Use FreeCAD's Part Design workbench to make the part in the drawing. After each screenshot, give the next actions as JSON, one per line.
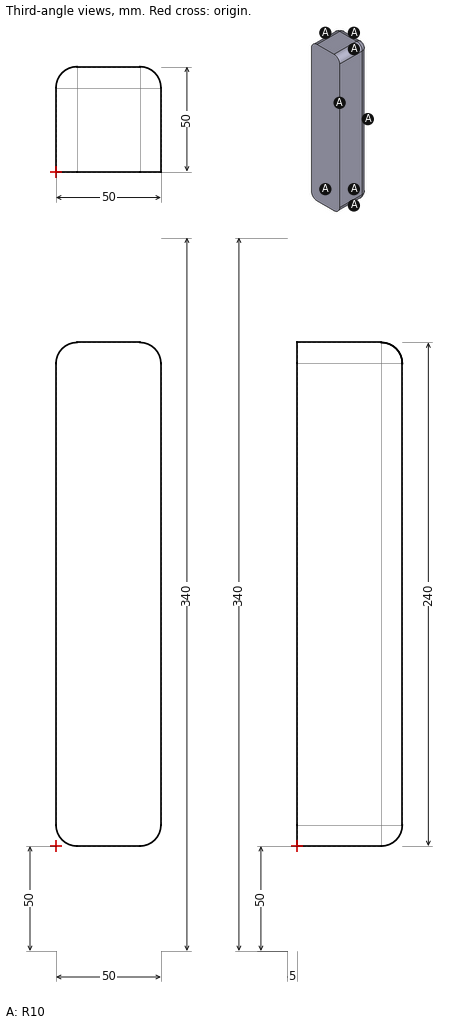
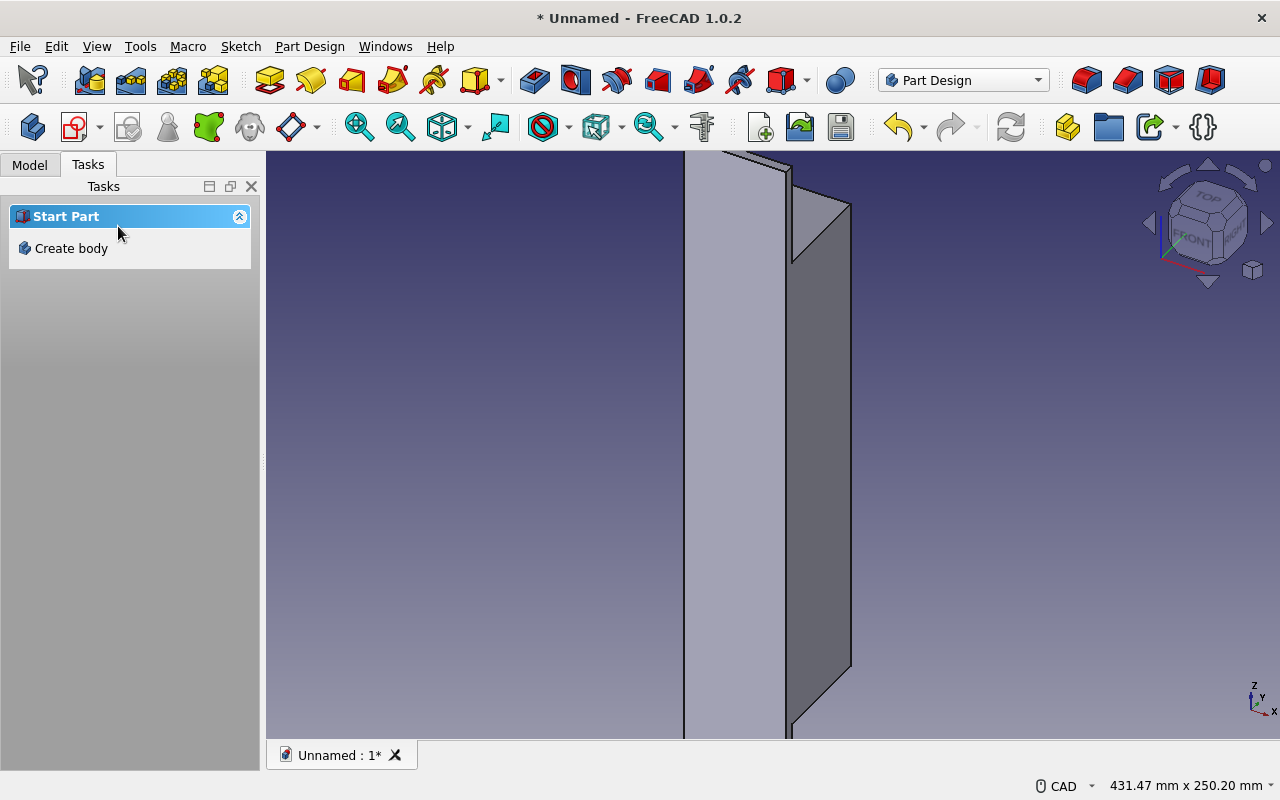
{"action": "left_click", "coordinate": [360, 128]}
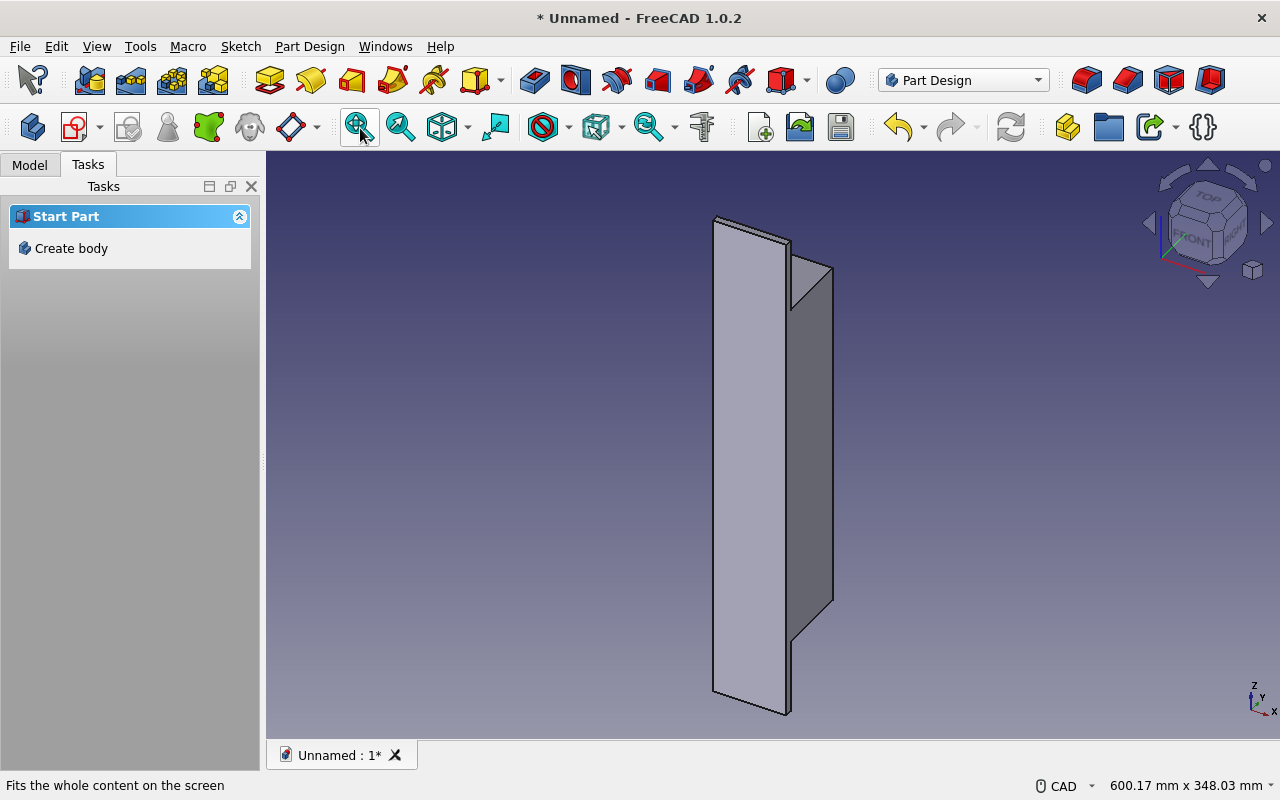
{"action": "left_click", "coordinate": [812, 288]}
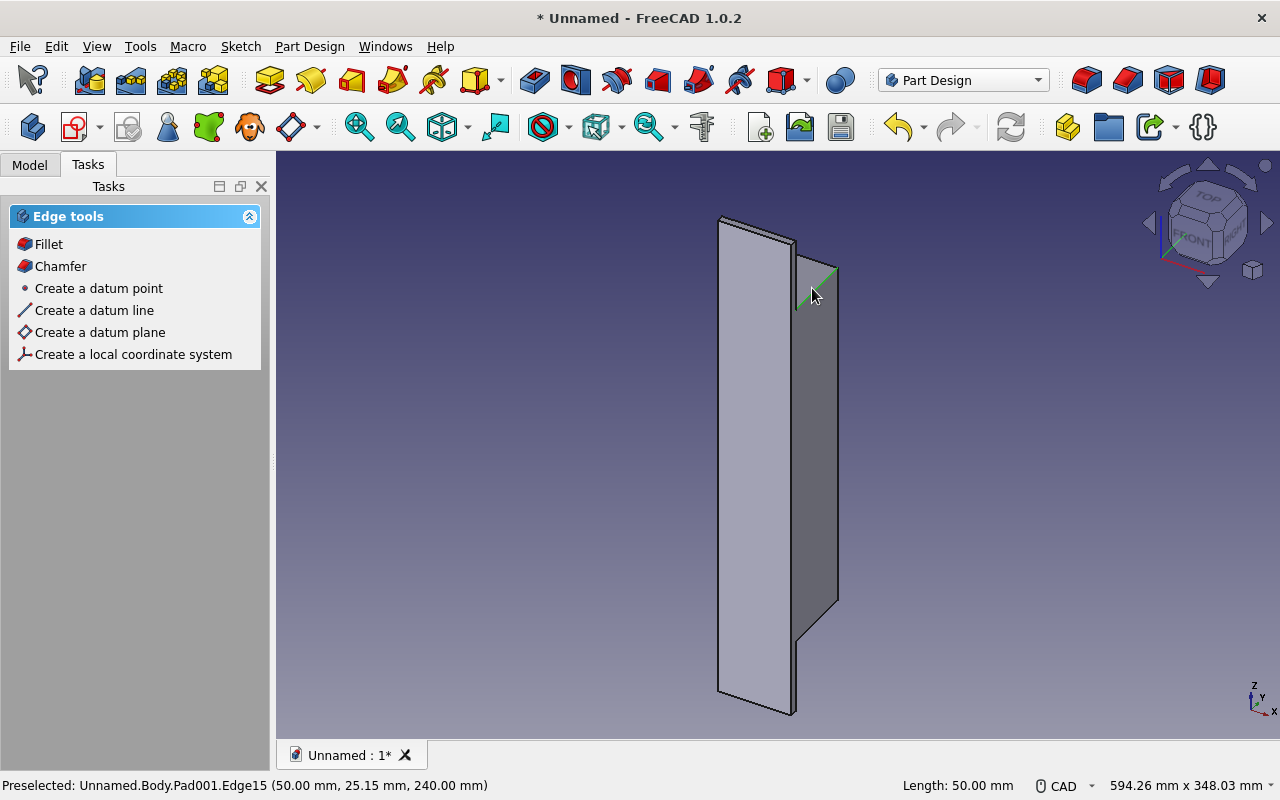
{"action": "key", "text": "0"}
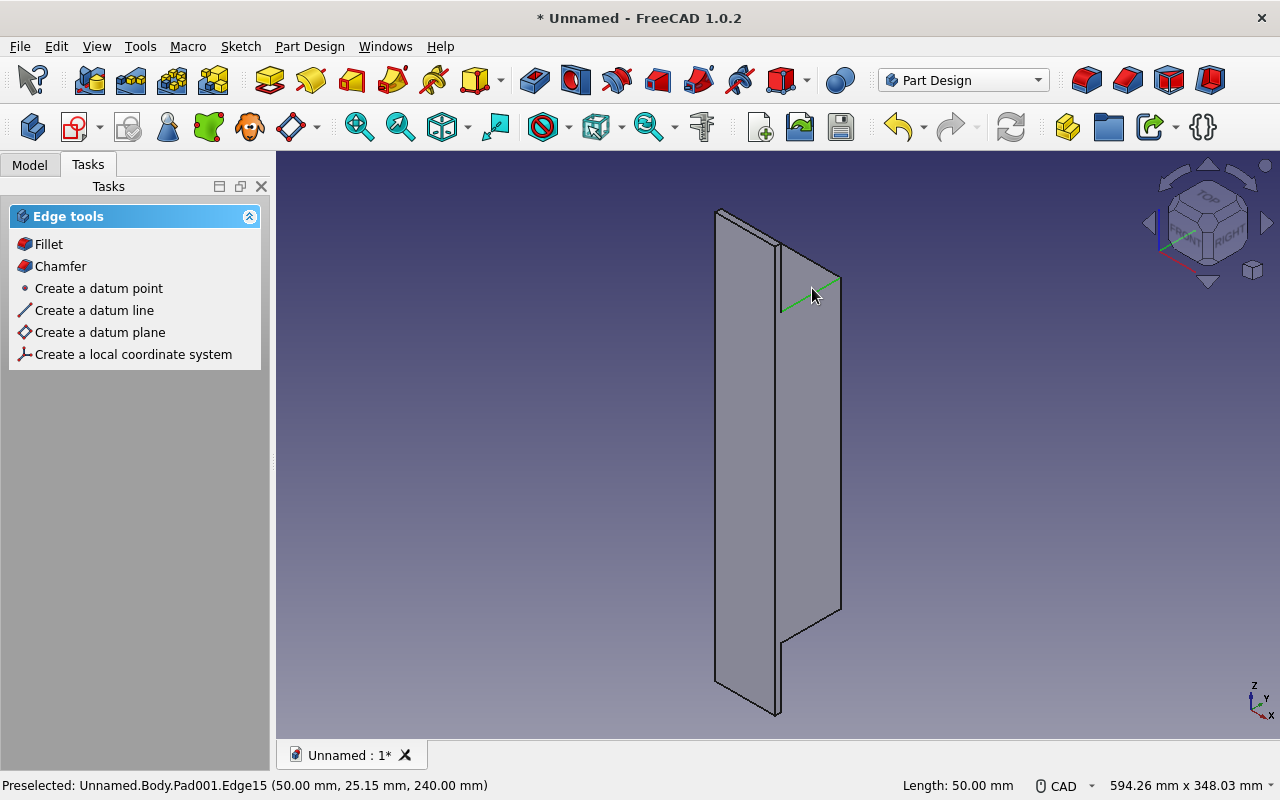
{"action": "key", "text": "2"}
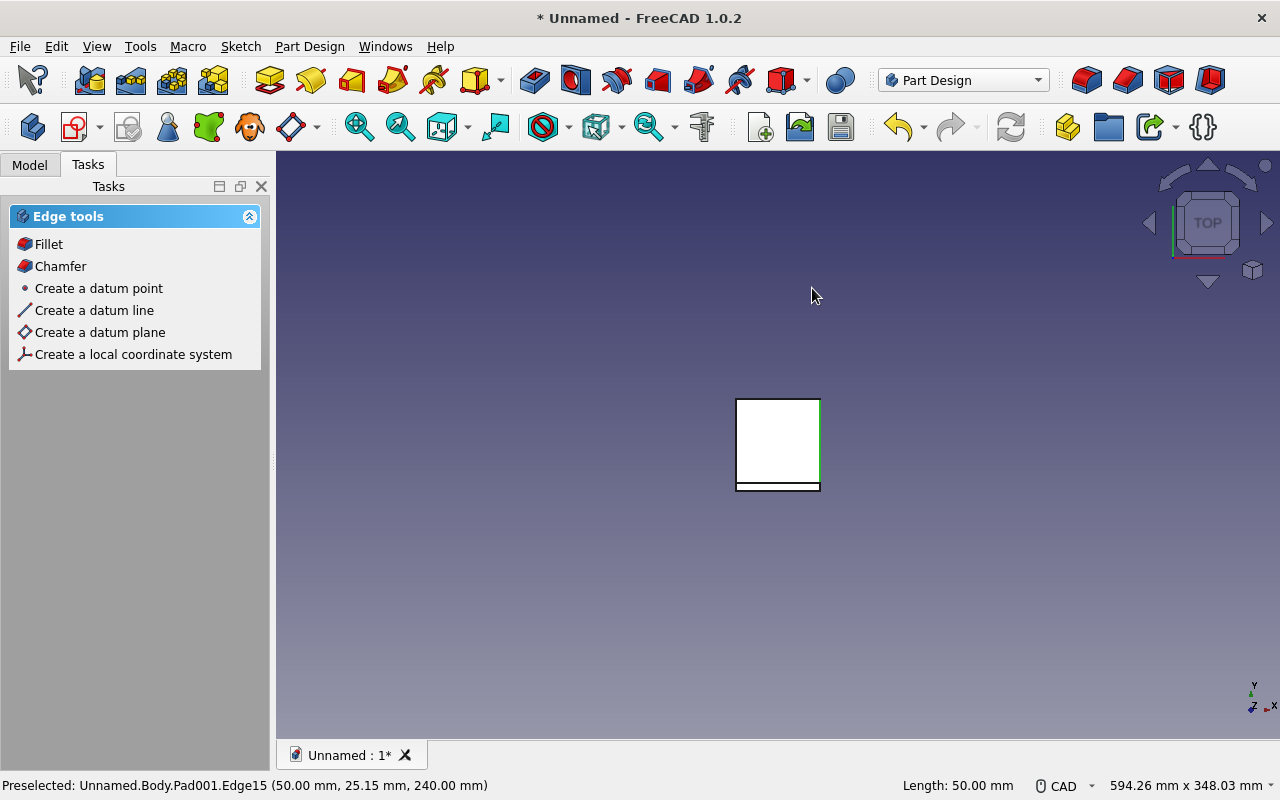
{"action": "left_click", "coordinate": [360, 128]}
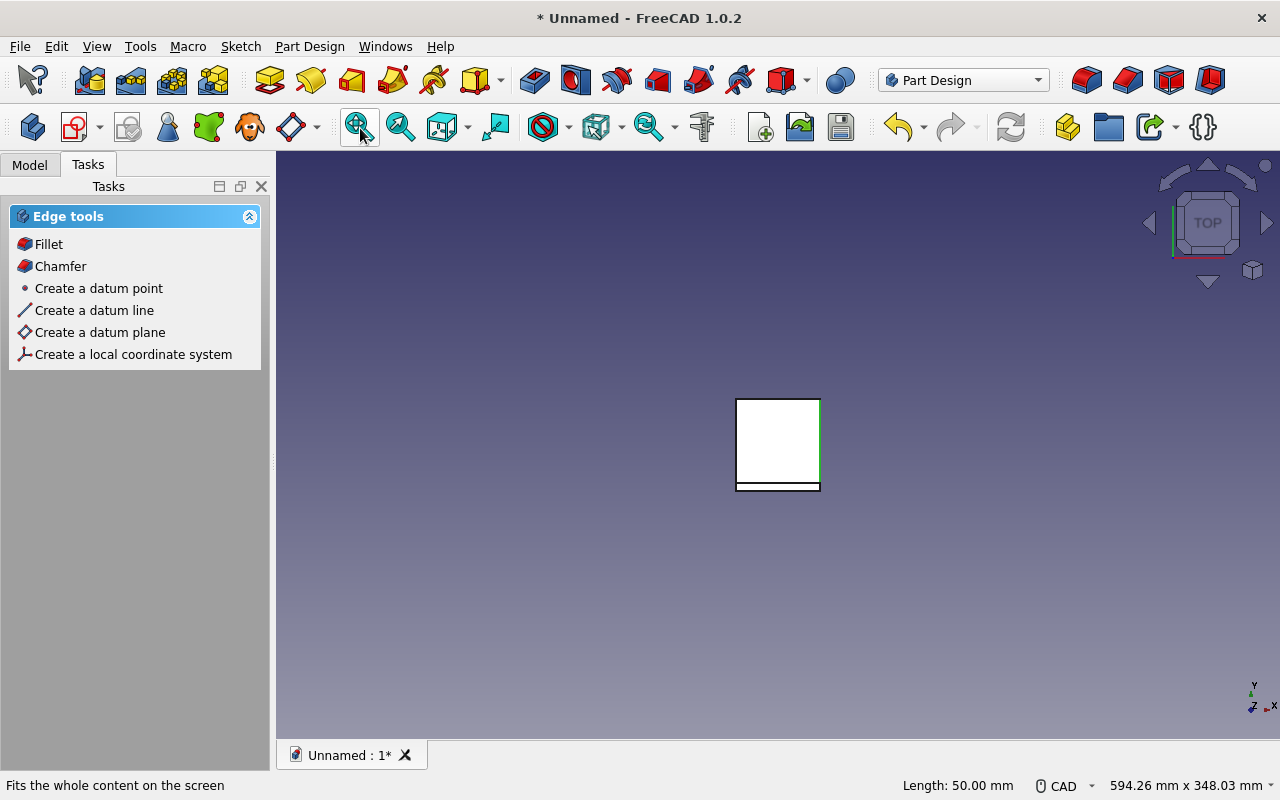
{"action": "left_click", "coordinate": [736, 440], "text": "ctrl"}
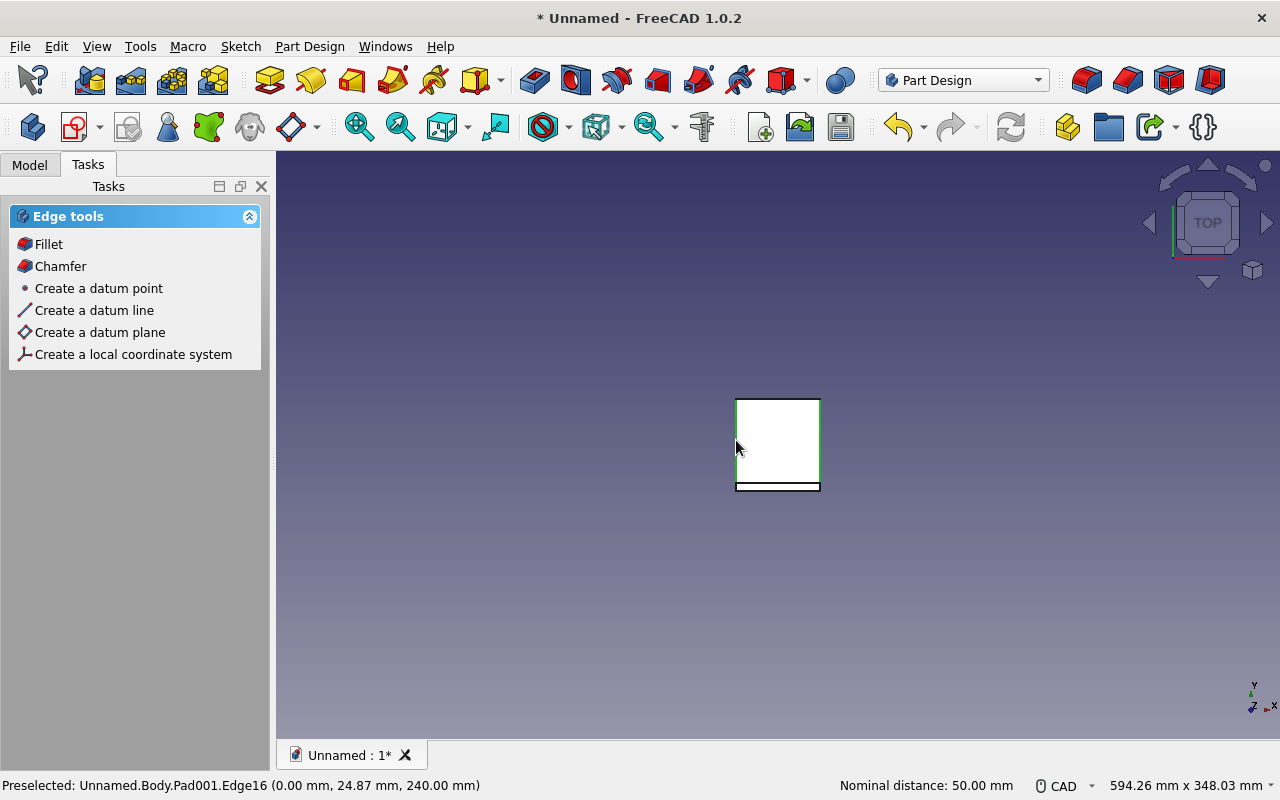
{"action": "key", "text": "1"}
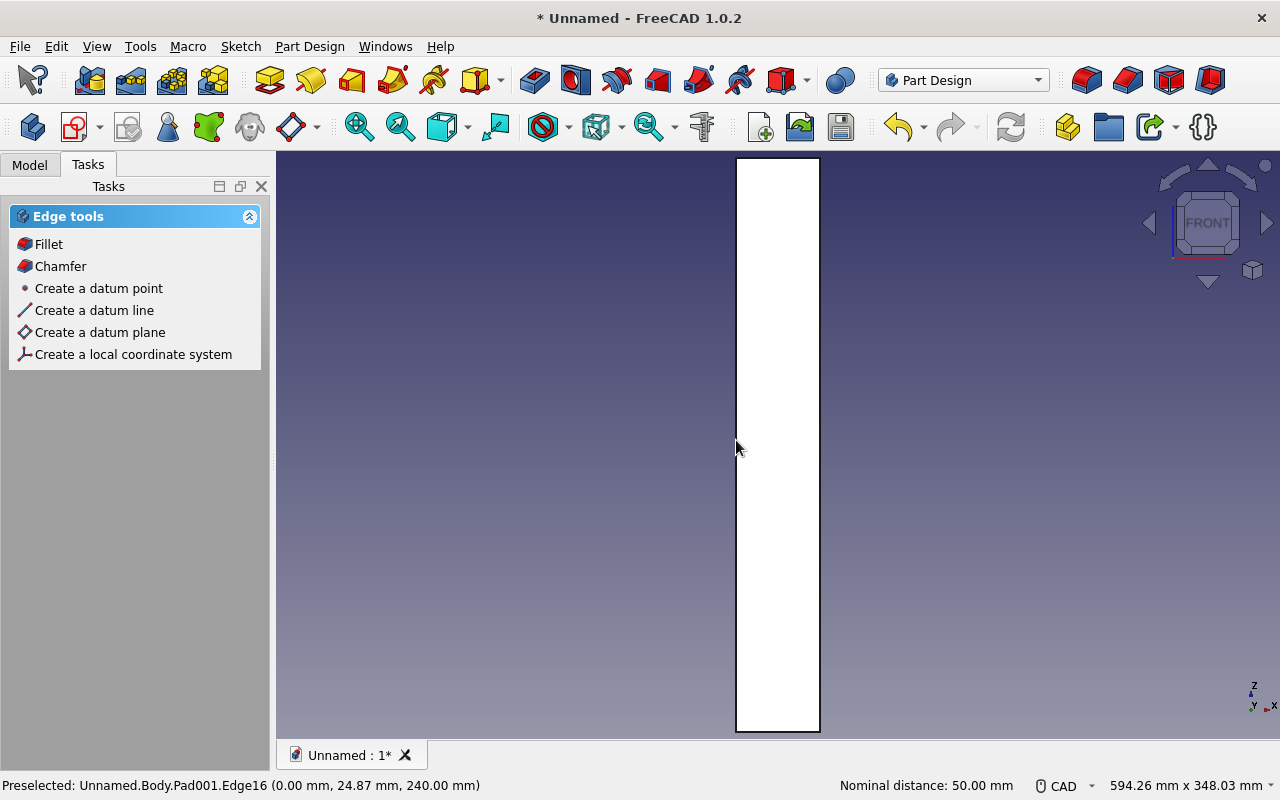
{"action": "key", "text": "3"}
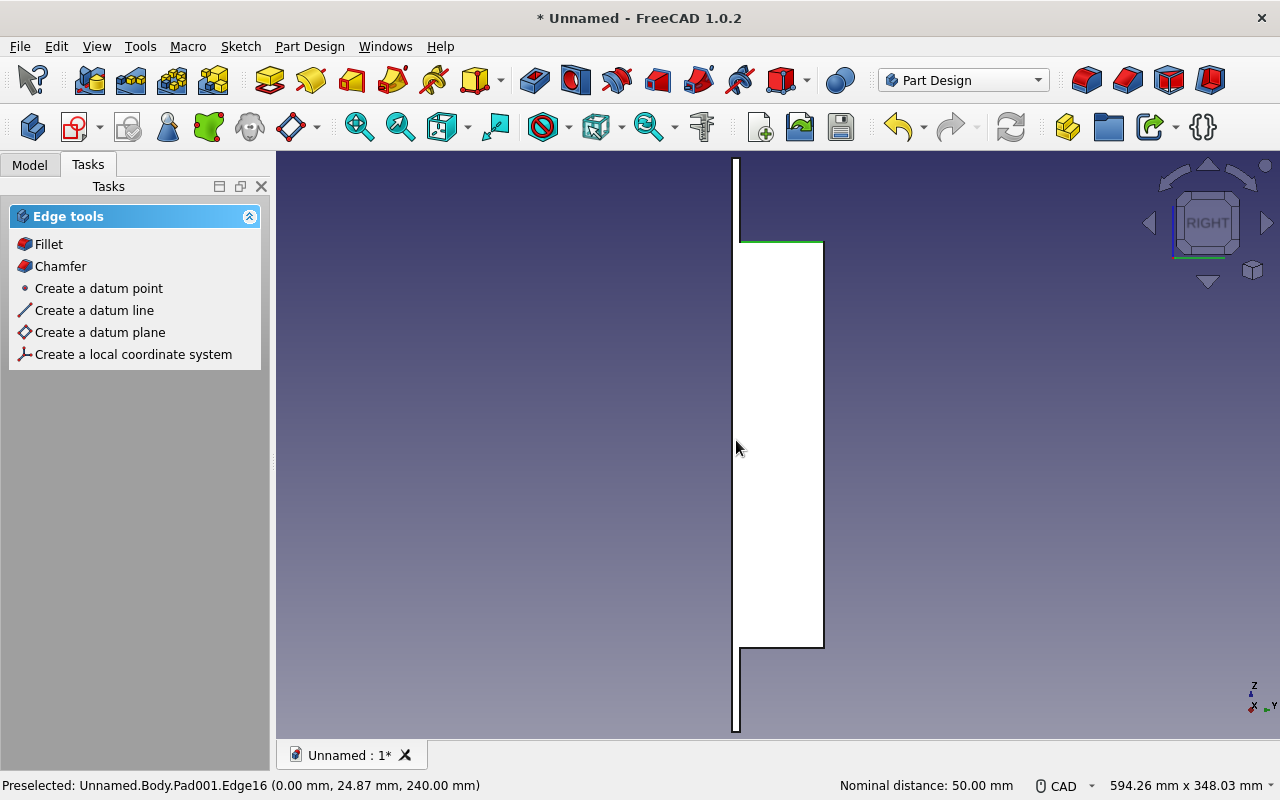
{"action": "left_click", "coordinate": [782, 647], "text": "ctrl"}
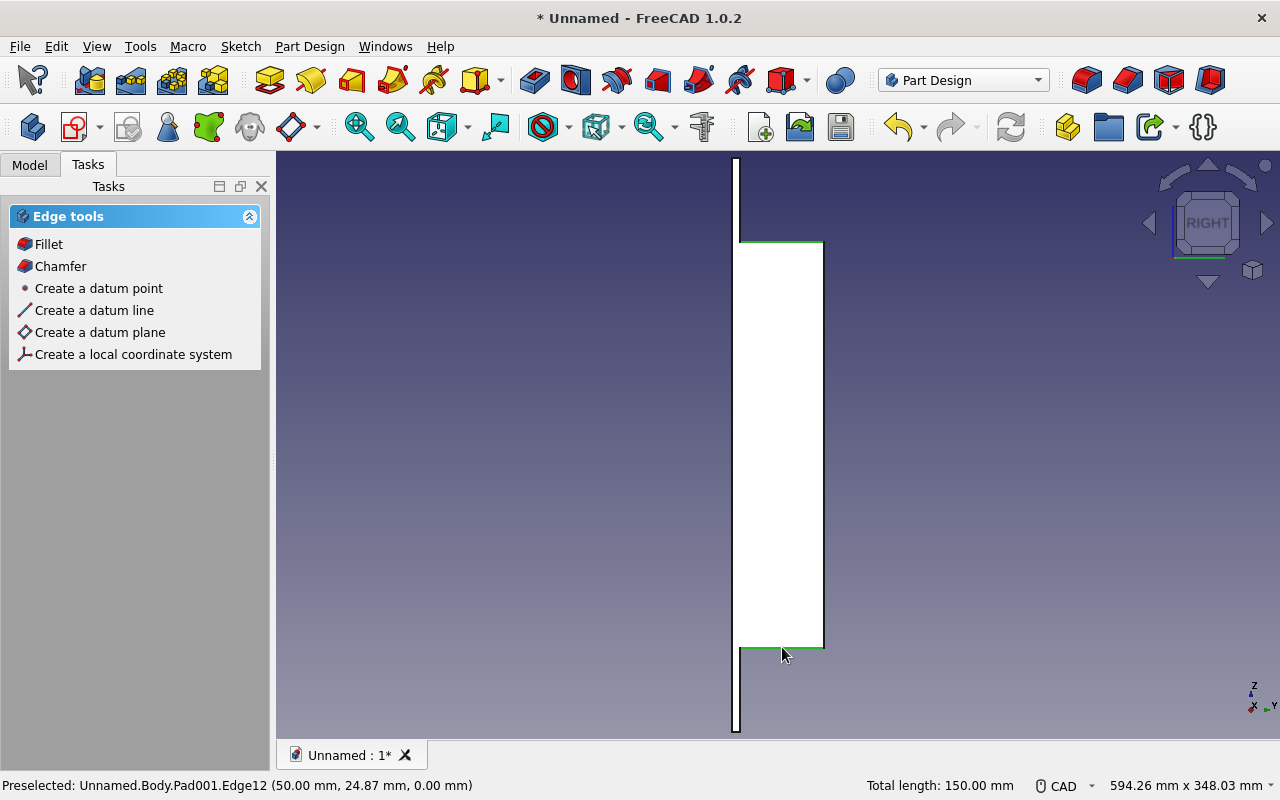
{"action": "key", "text": "5"}